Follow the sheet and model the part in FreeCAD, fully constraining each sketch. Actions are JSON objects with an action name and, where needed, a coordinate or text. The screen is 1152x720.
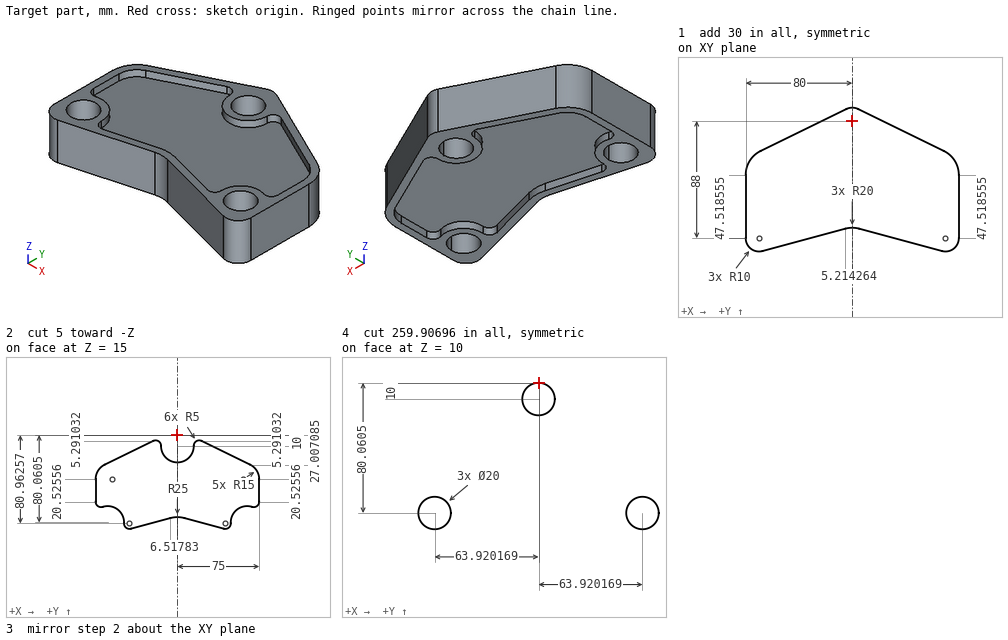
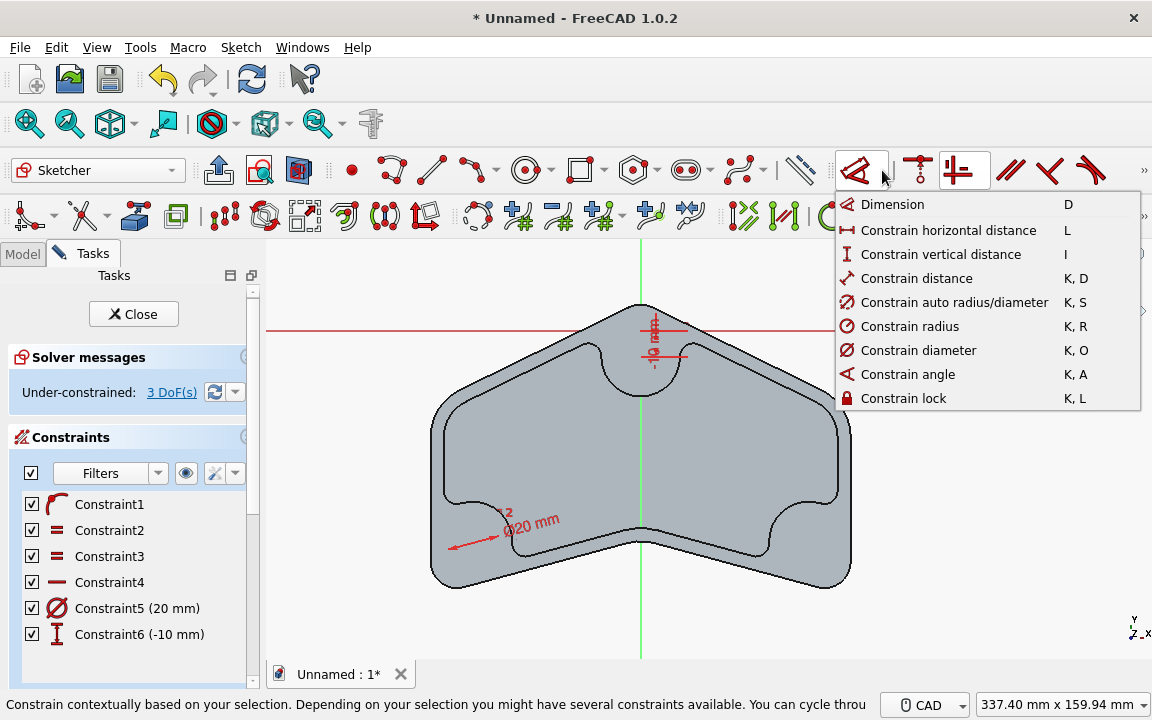
{"action": "left_click", "coordinate": [988, 254]}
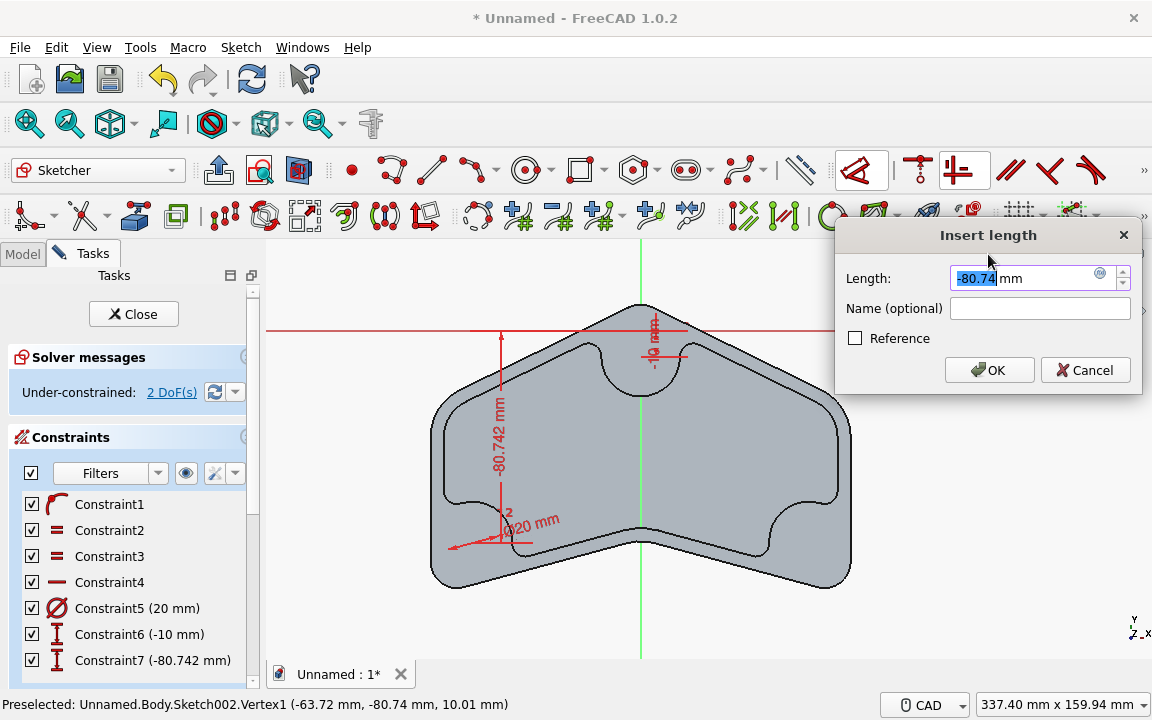
{"action": "type", "text": "-80.0605"}
{"action": "key", "text": "Return"}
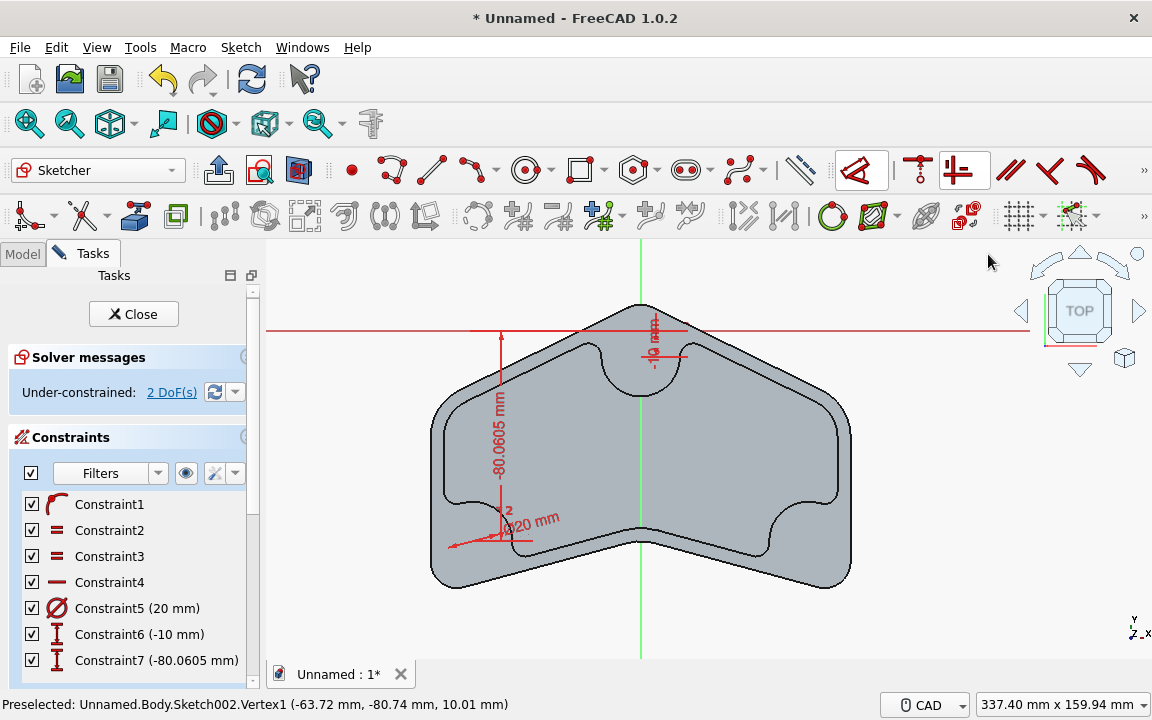
{"action": "left_click", "coordinate": [473, 541]}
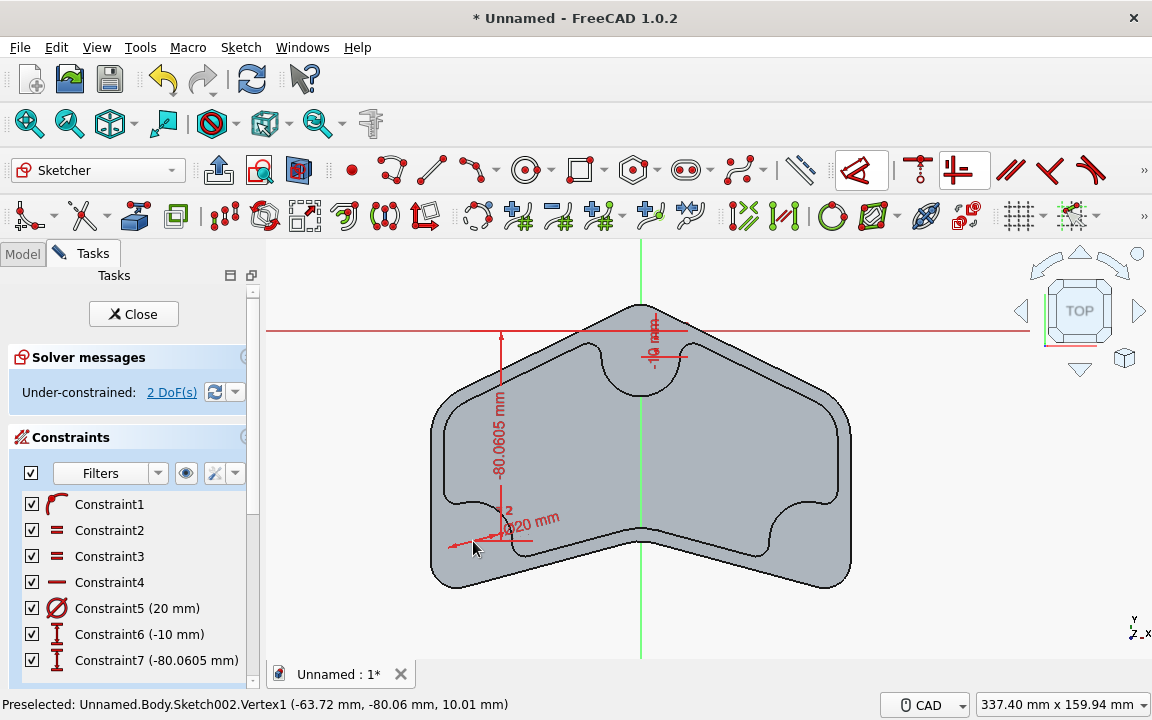
{"action": "left_click", "coordinate": [882, 170]}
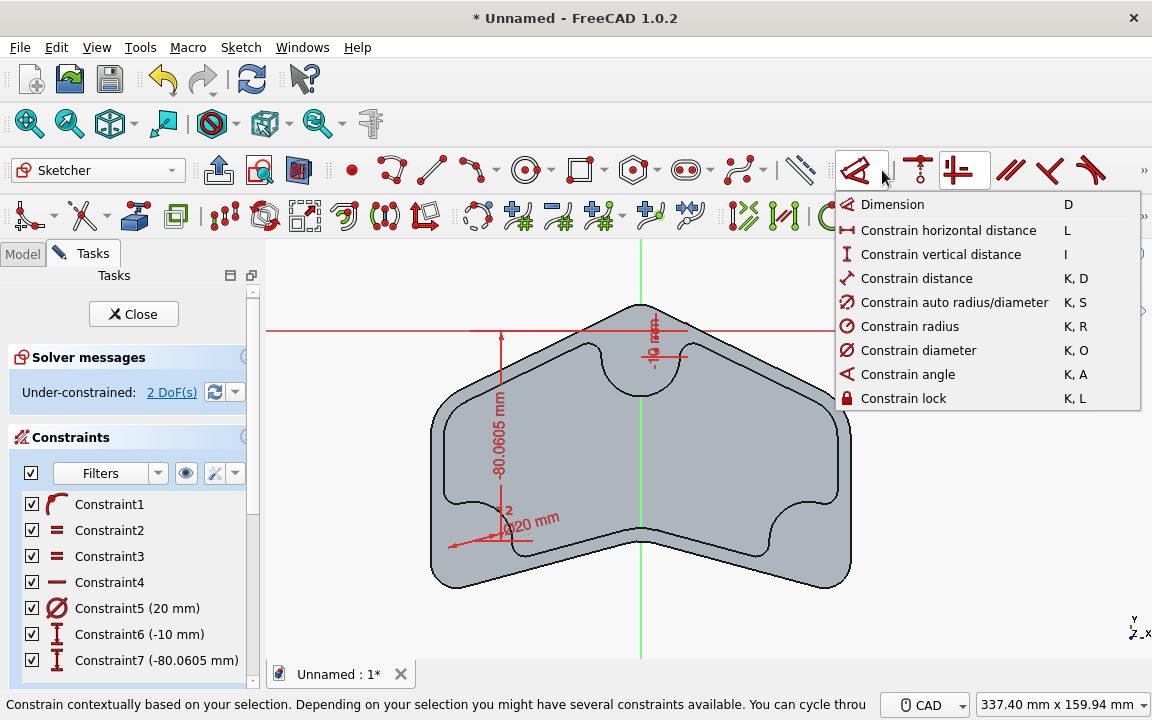
{"action": "left_click", "coordinate": [988, 230]}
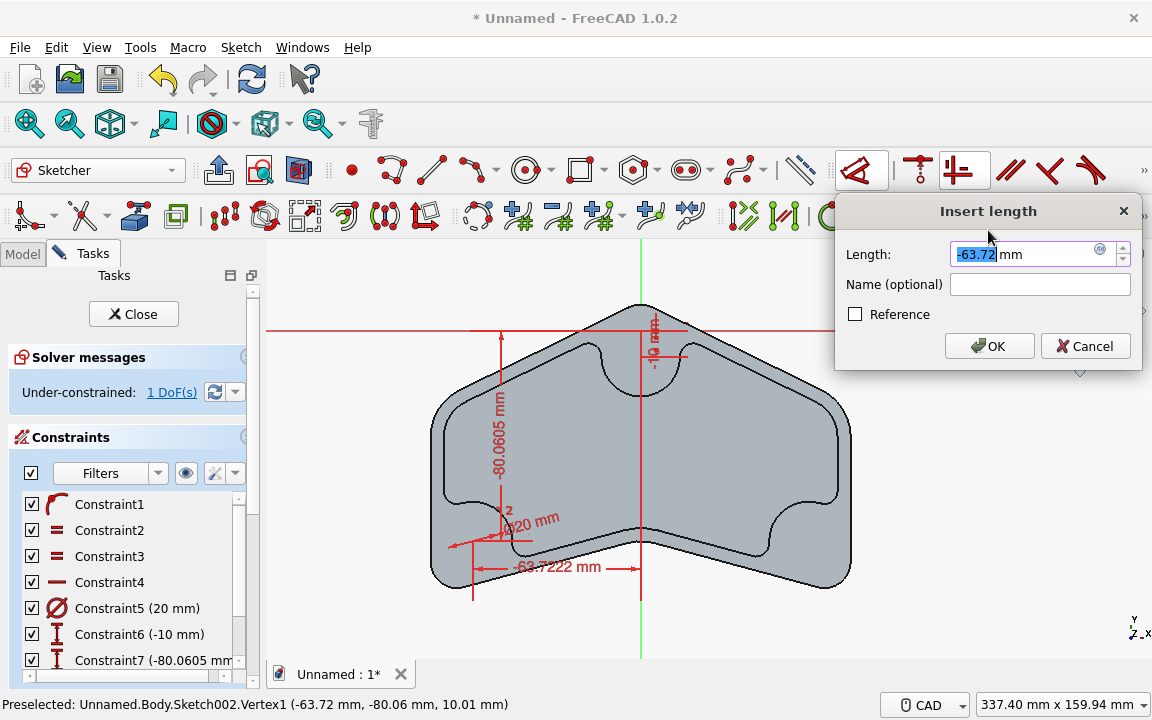
{"action": "type", "text": "-63.920169"}
{"action": "key", "text": "Return"}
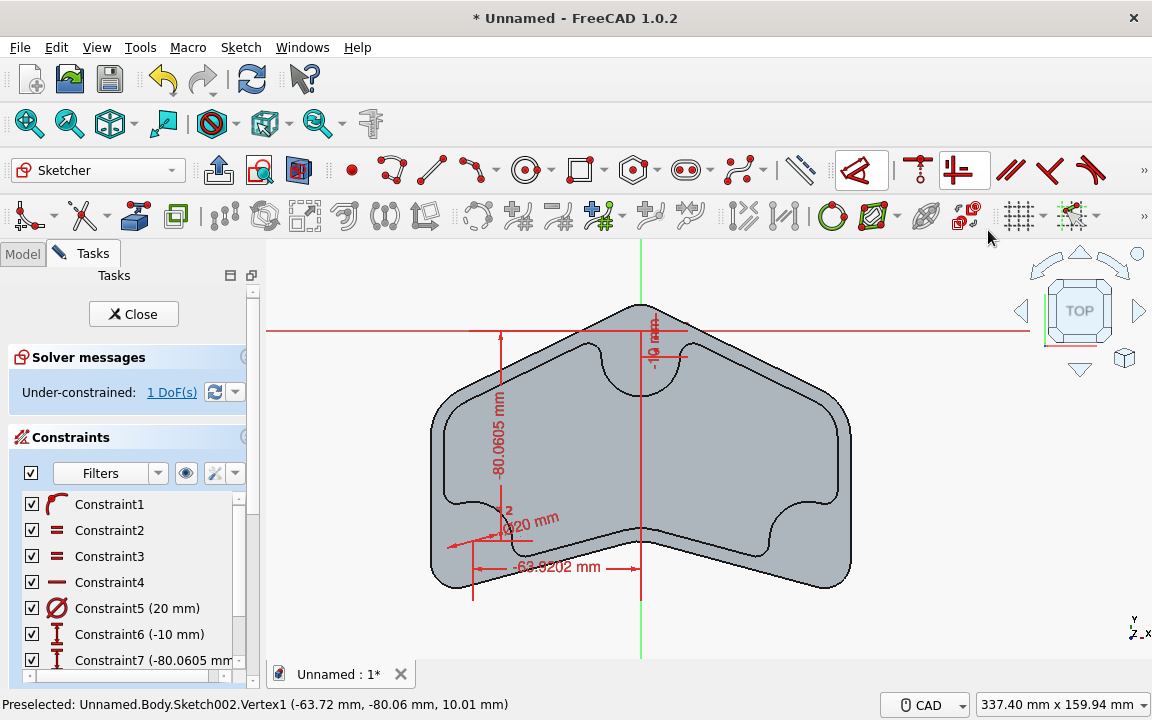
{"action": "left_click", "coordinate": [808, 541]}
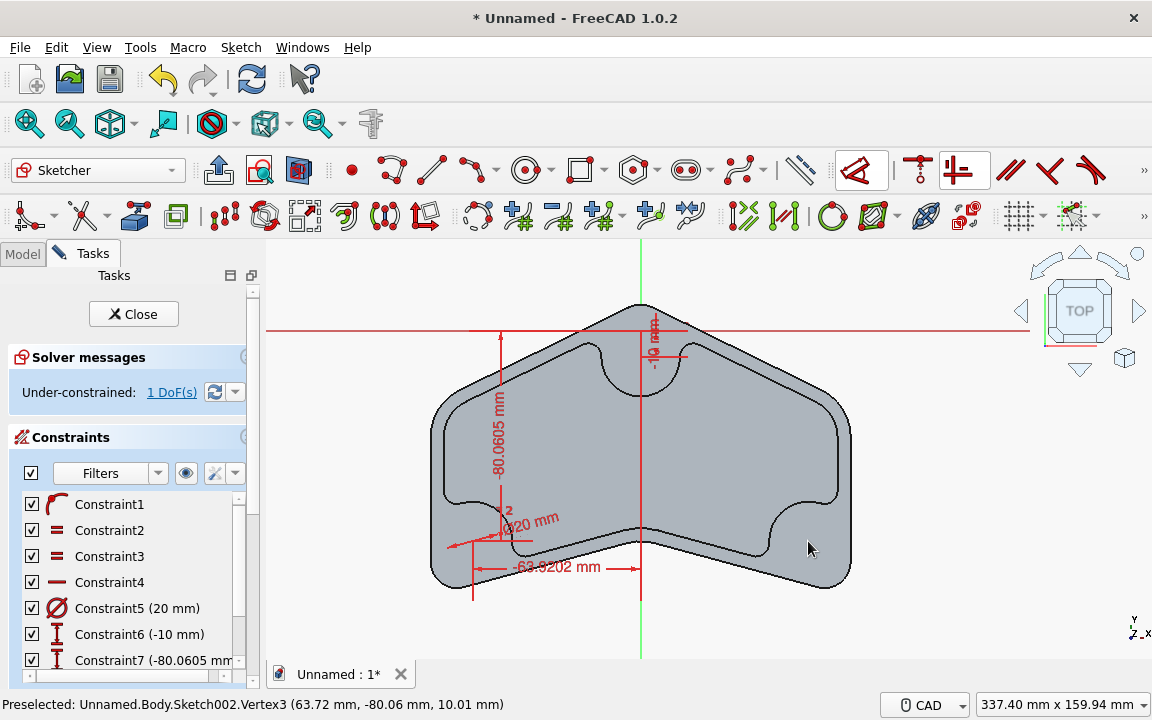
{"action": "left_click", "coordinate": [882, 170]}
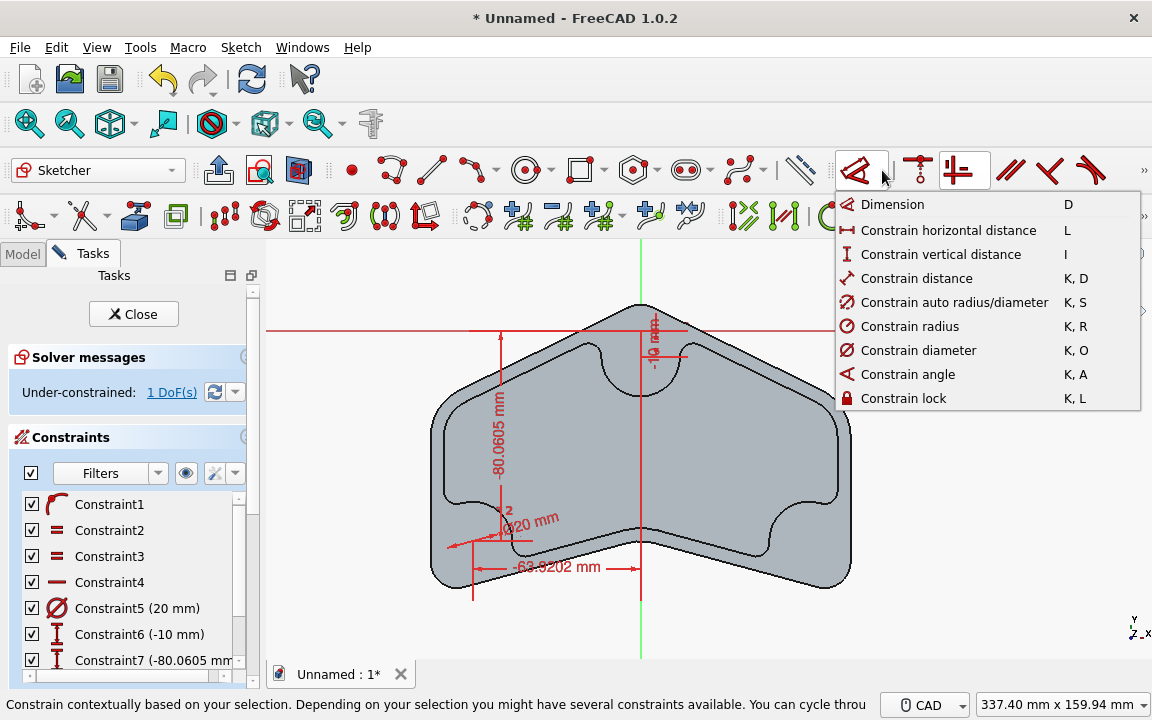
{"action": "left_click", "coordinate": [988, 230]}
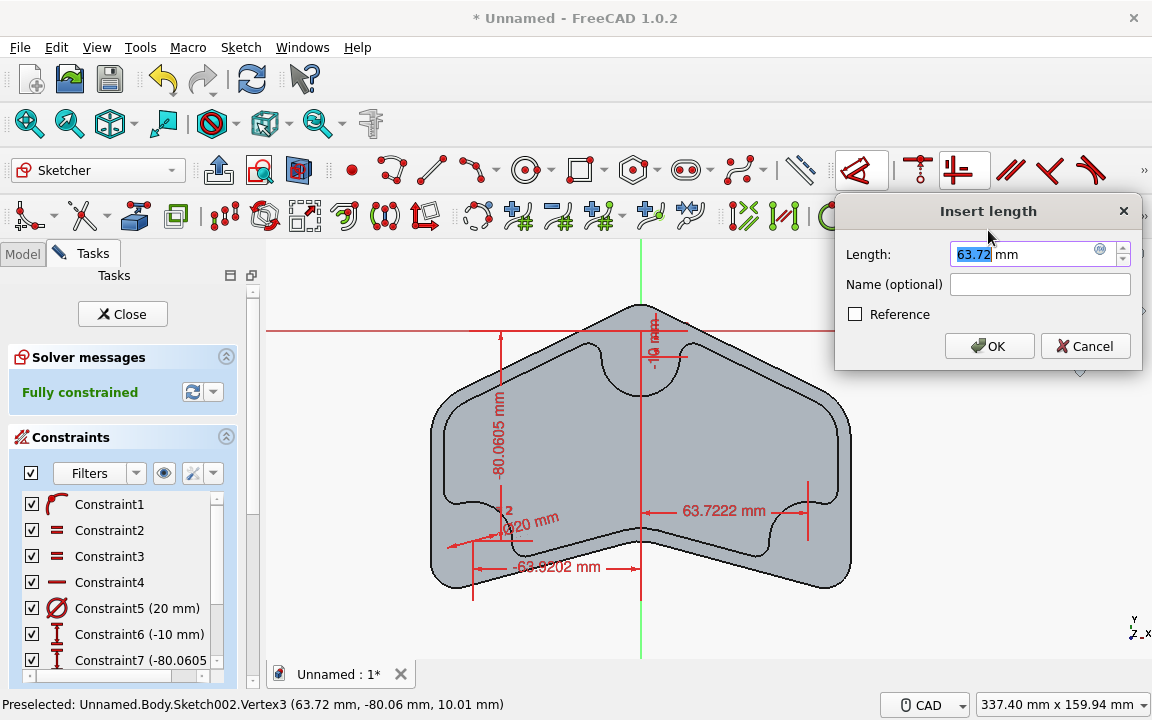
{"action": "type", "text": "63.920169"}
{"action": "key", "text": "Return"}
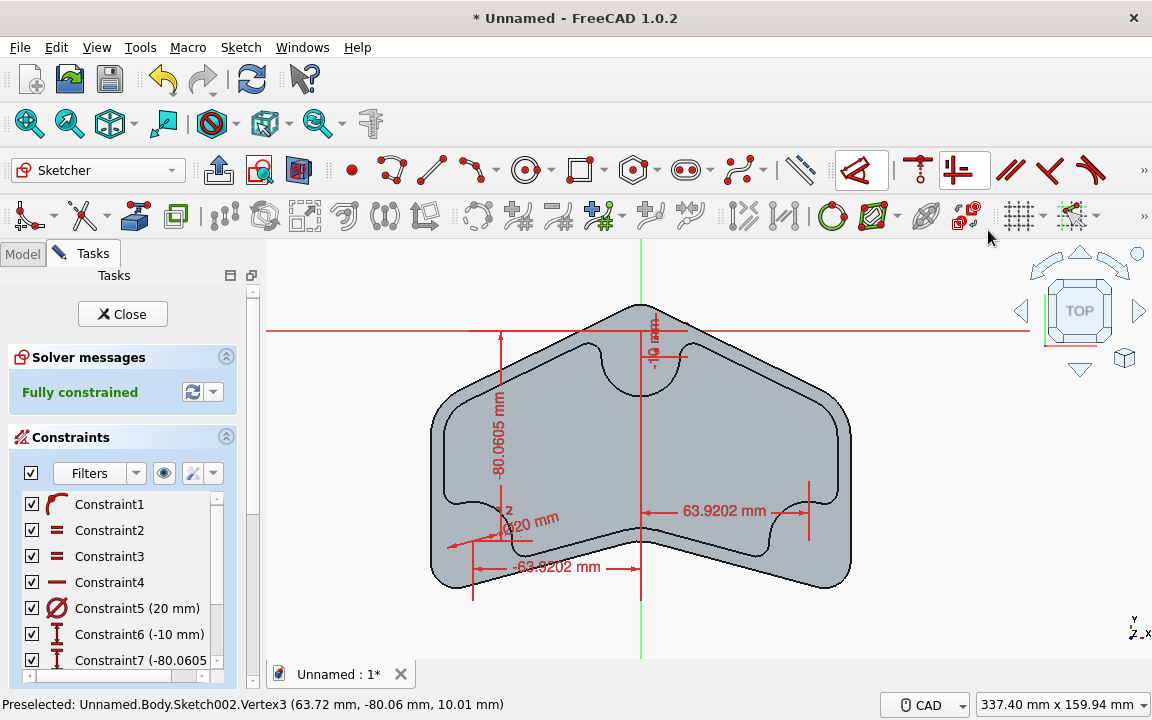
{"action": "left_click", "coordinate": [123, 314]}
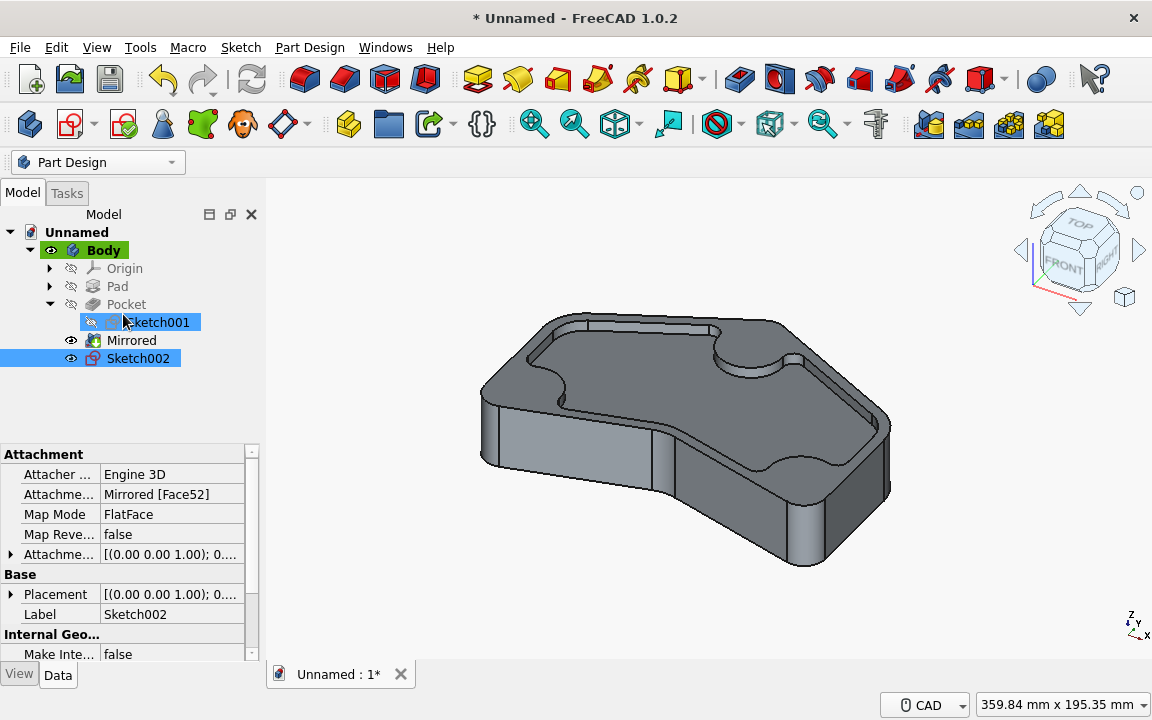
{"action": "left_click", "coordinate": [740, 80]}